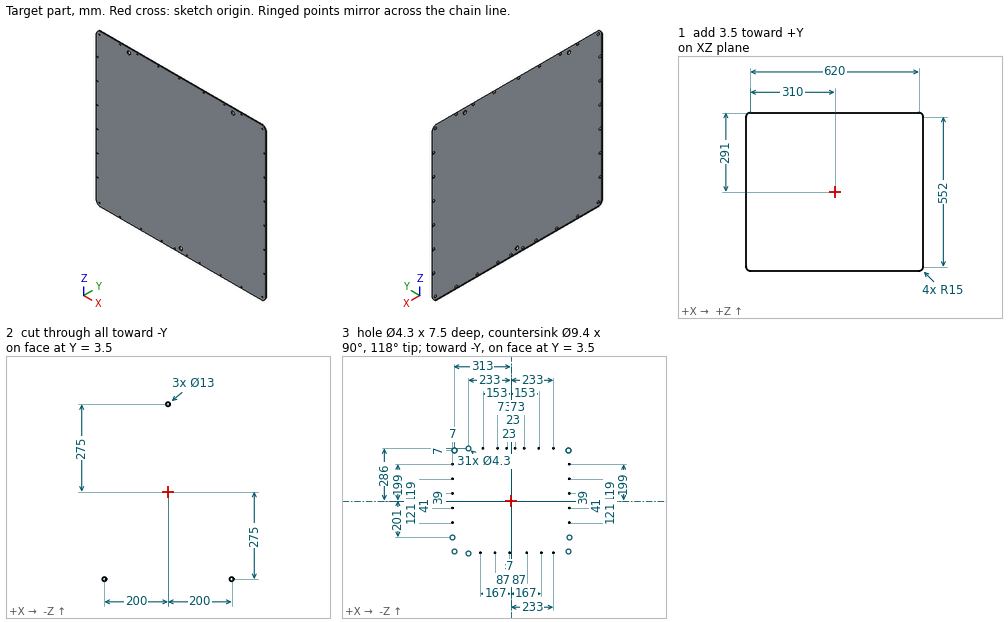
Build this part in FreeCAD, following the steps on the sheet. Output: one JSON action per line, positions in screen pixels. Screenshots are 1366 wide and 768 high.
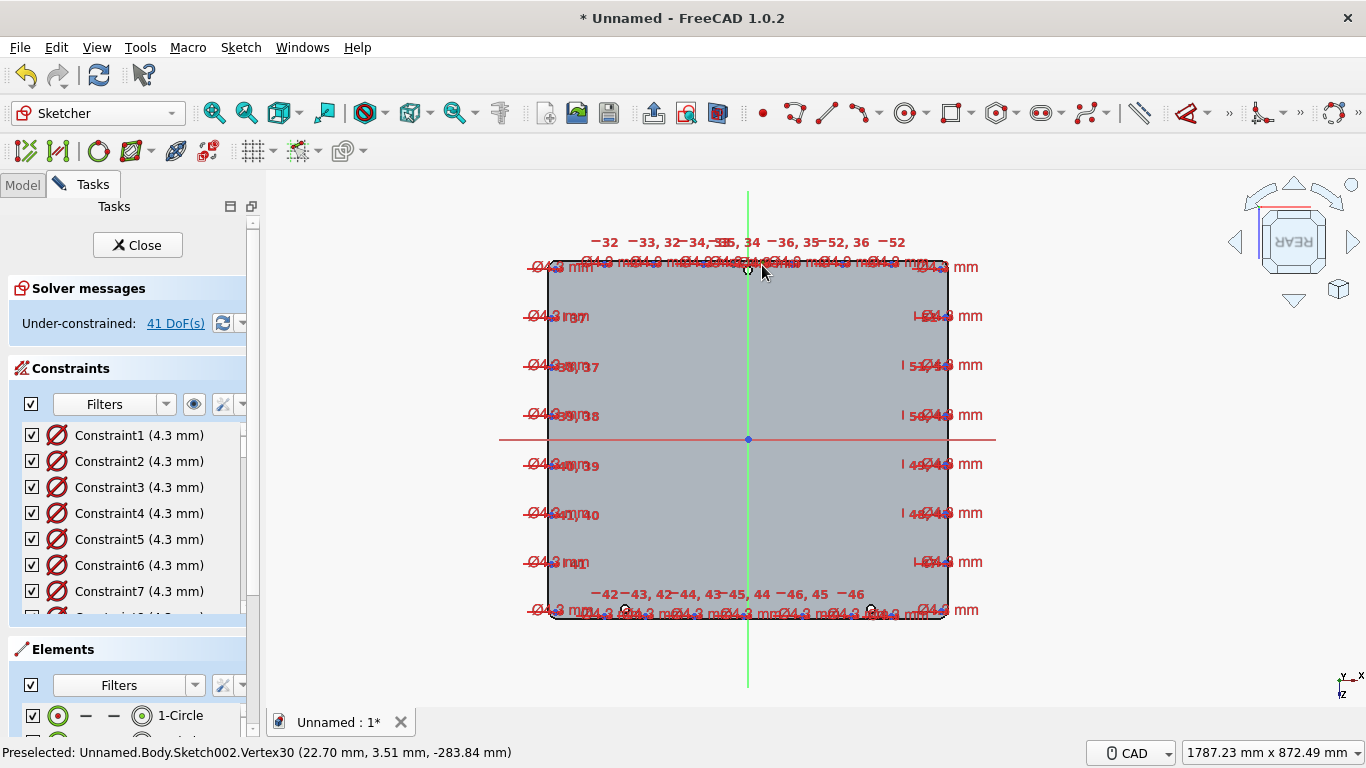
{"action": "key", "text": "h"}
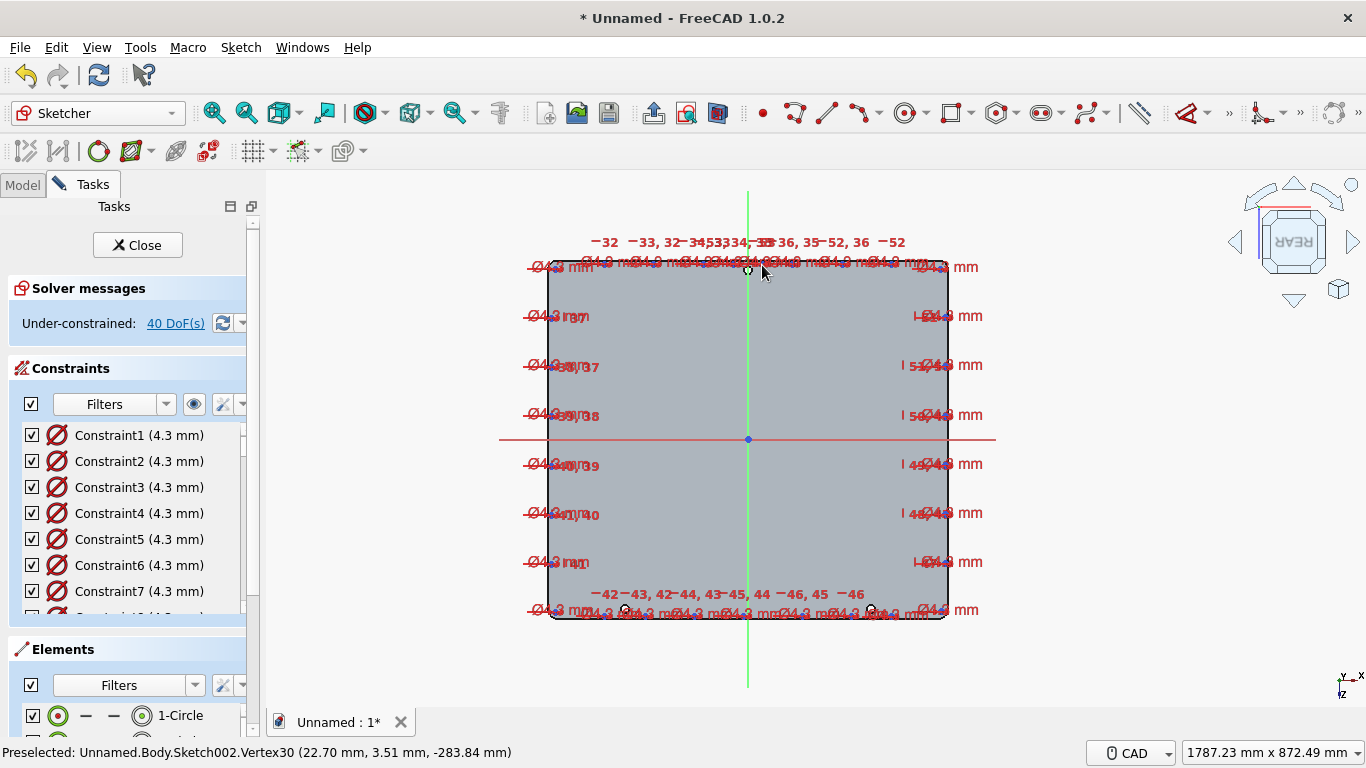
{"action": "left_click", "coordinate": [851, 616]}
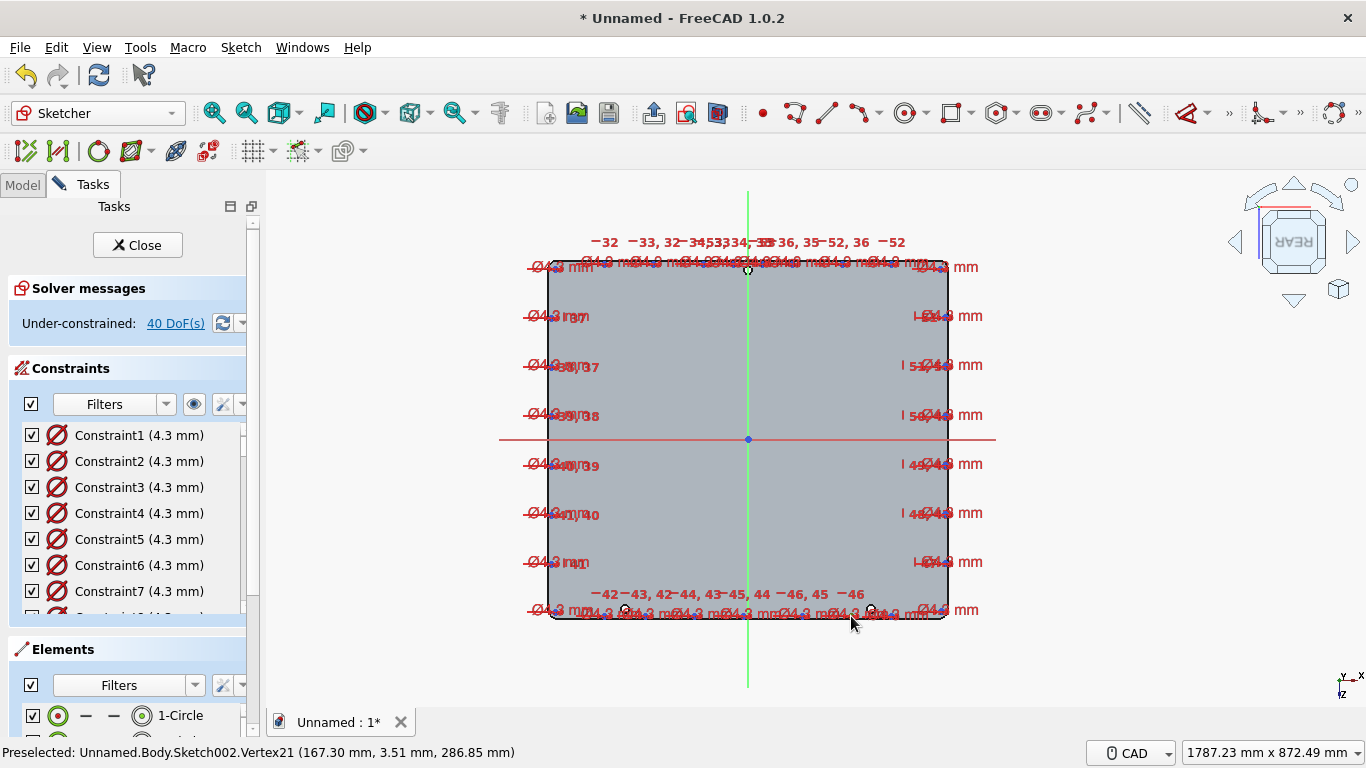
{"action": "left_click", "coordinate": [891, 617]}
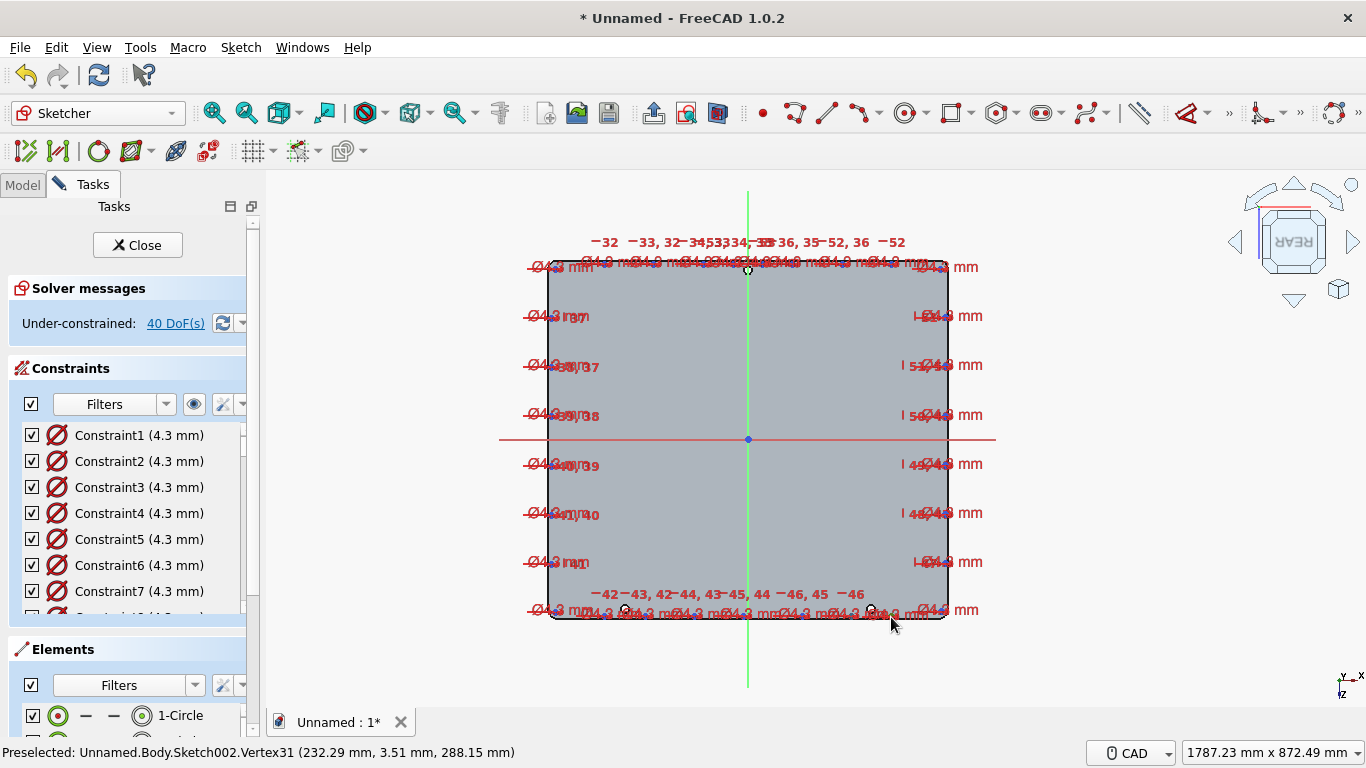
{"action": "key", "text": "h"}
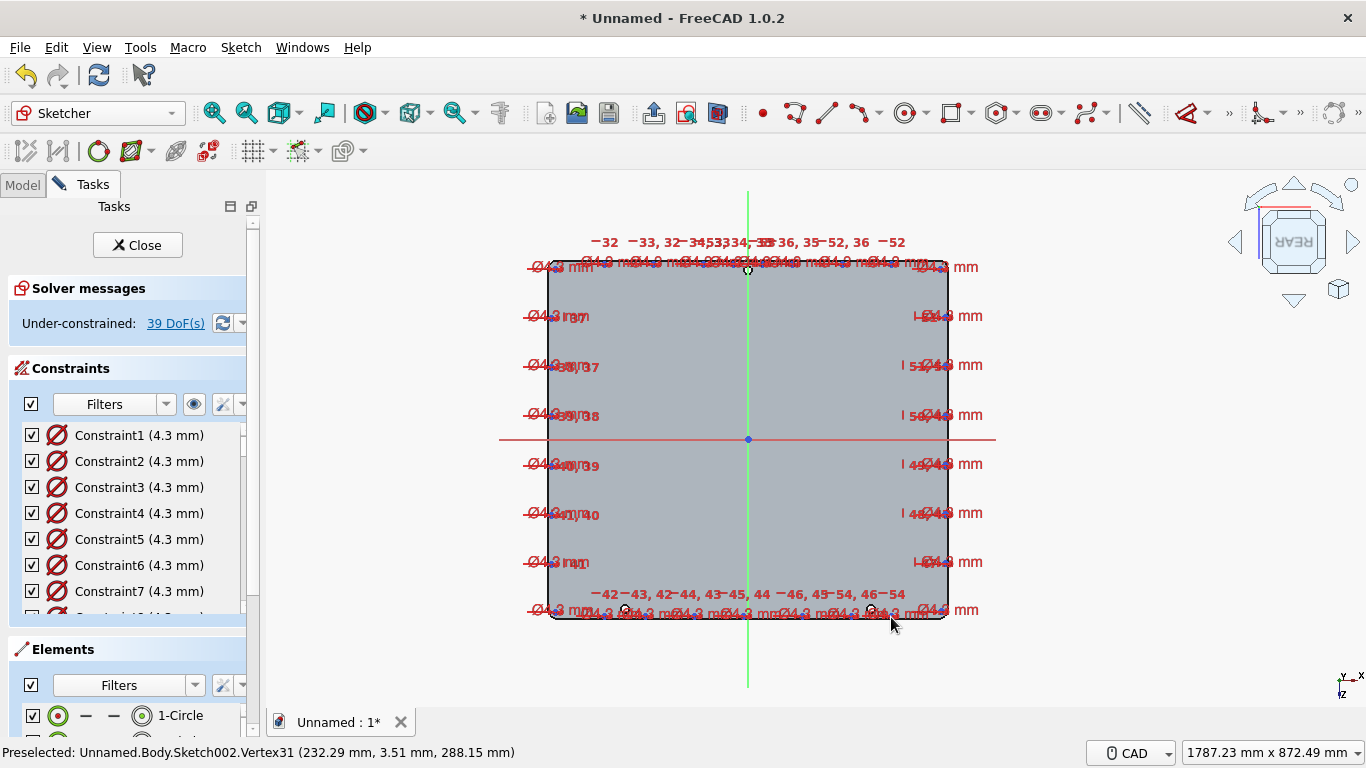
{"action": "left_click", "coordinate": [556, 269]}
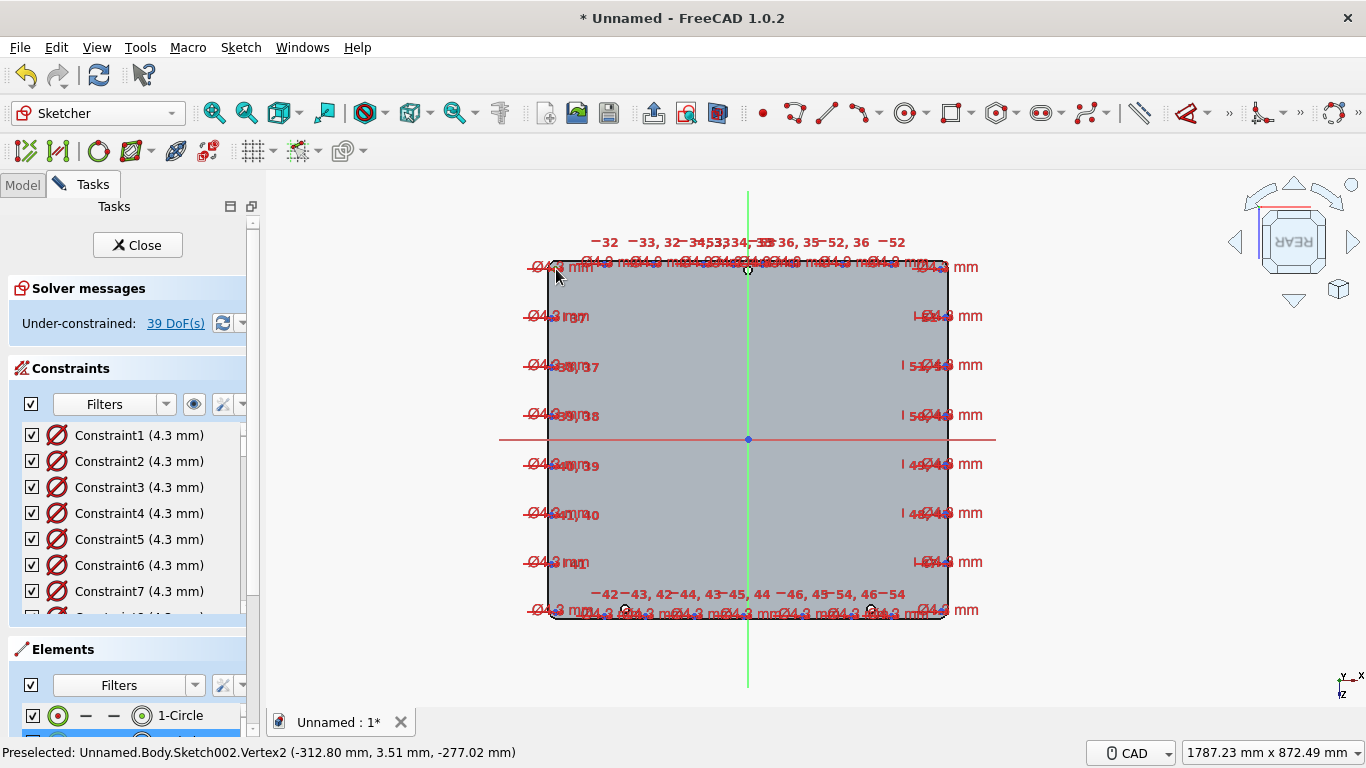
{"action": "left_click", "coordinate": [941, 269]}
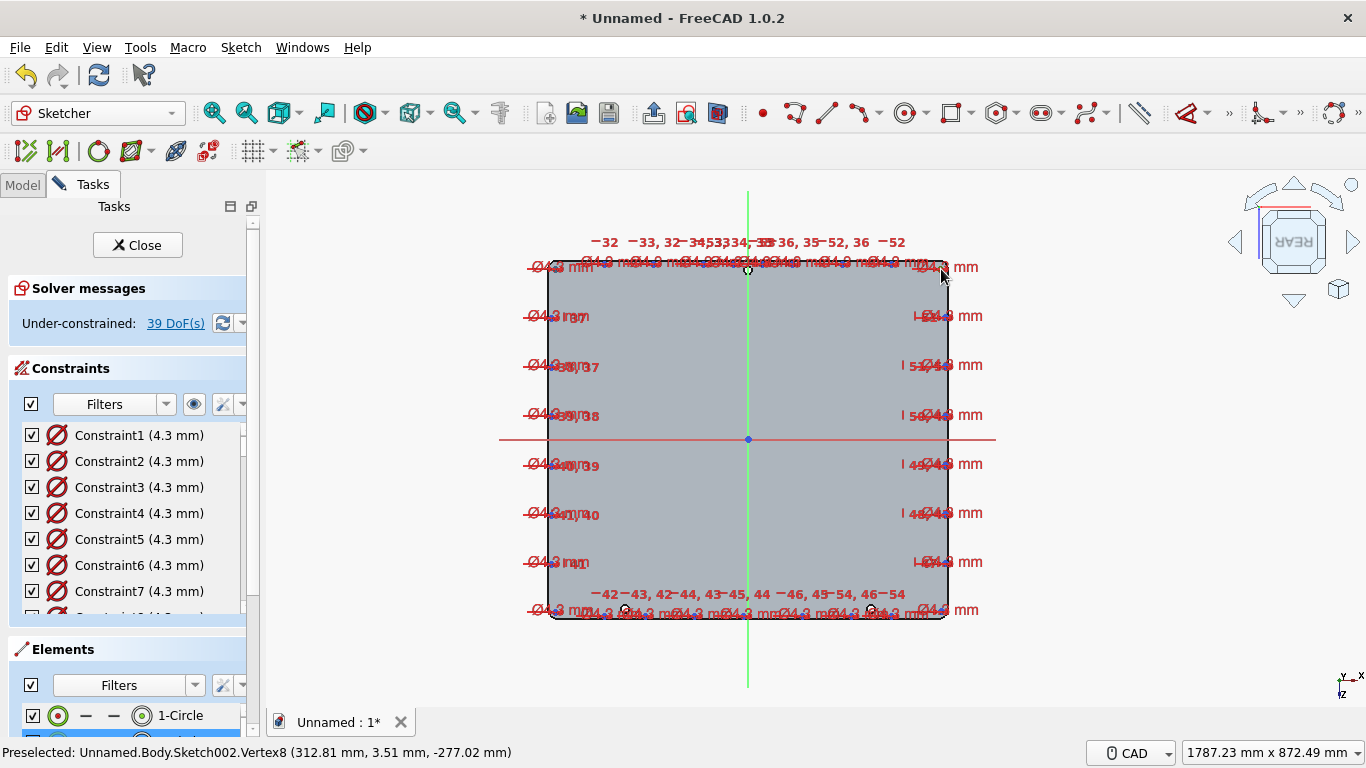
{"action": "left_click", "coordinate": [748, 576]}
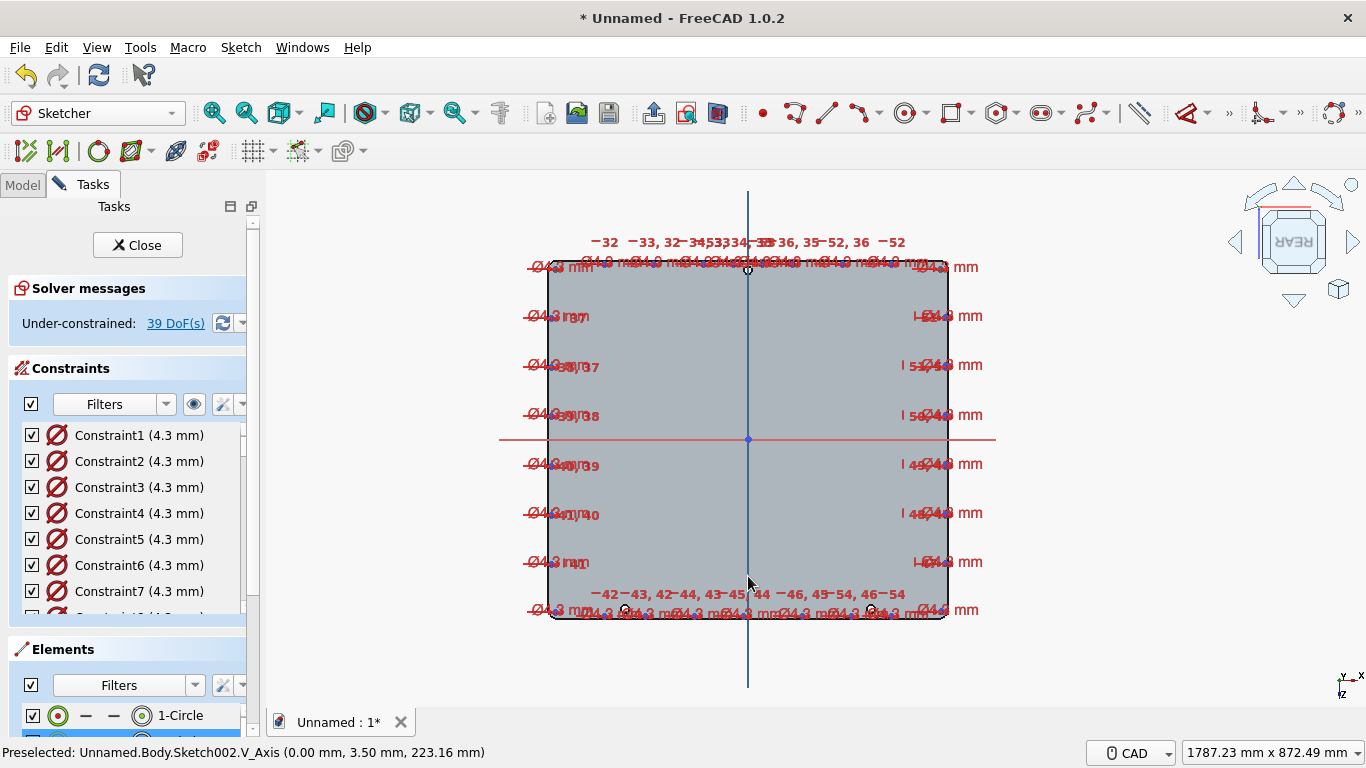
{"action": "key", "text": "s"}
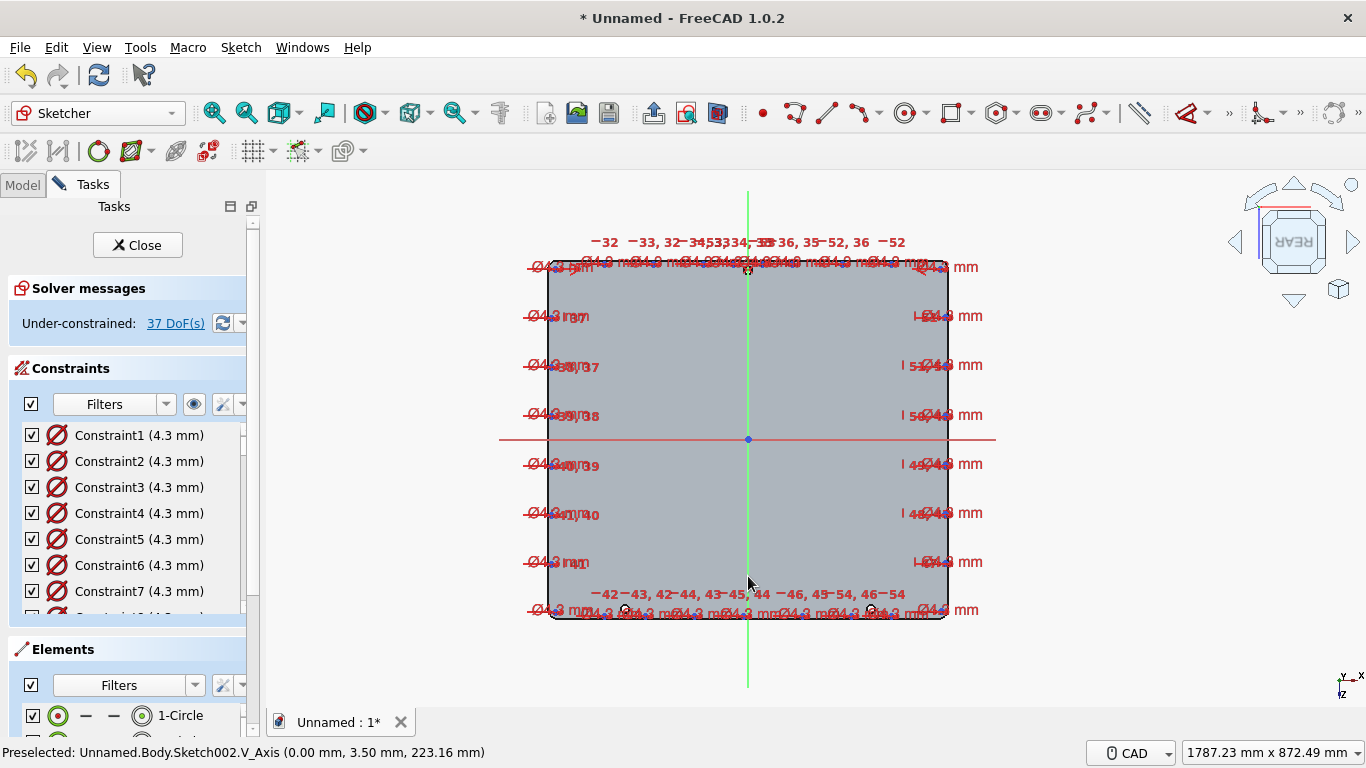
{"action": "left_click", "coordinate": [556, 269]}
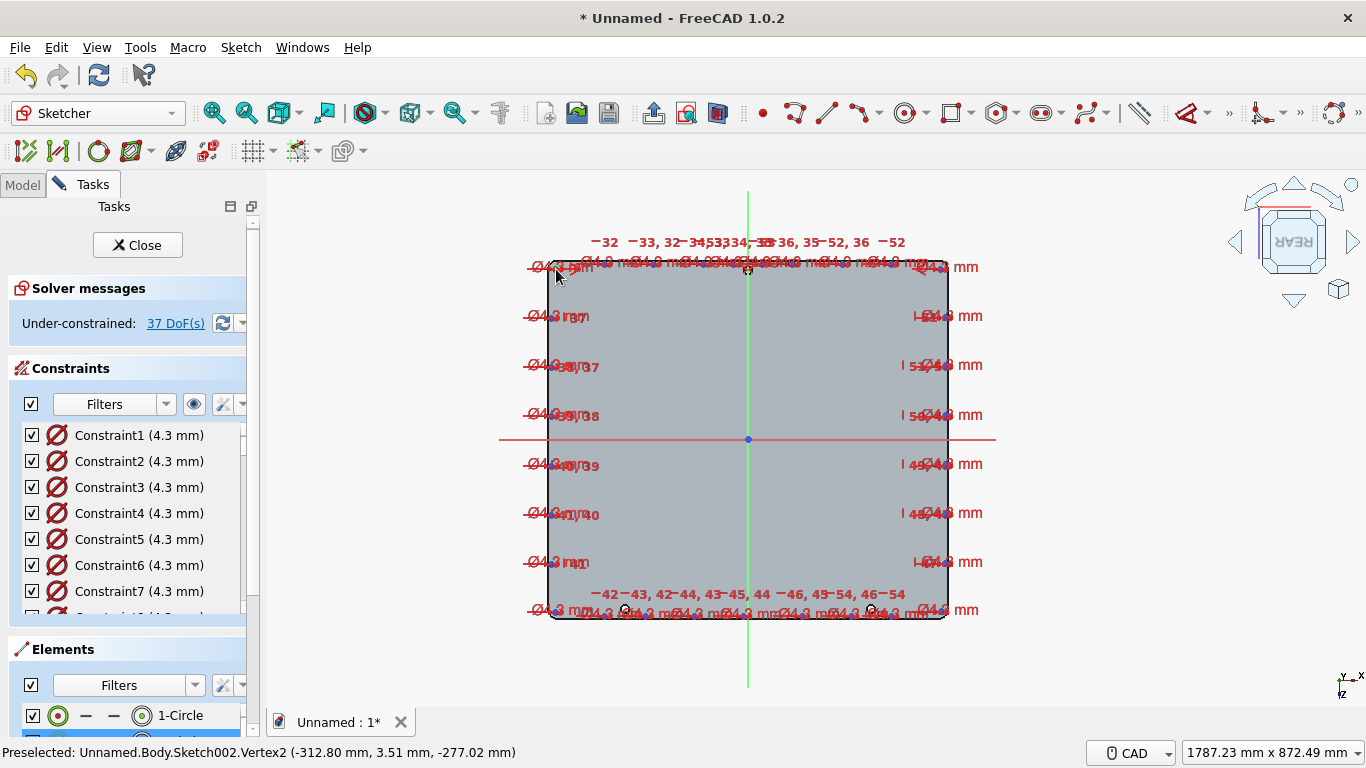
{"action": "left_click", "coordinate": [556, 612]}